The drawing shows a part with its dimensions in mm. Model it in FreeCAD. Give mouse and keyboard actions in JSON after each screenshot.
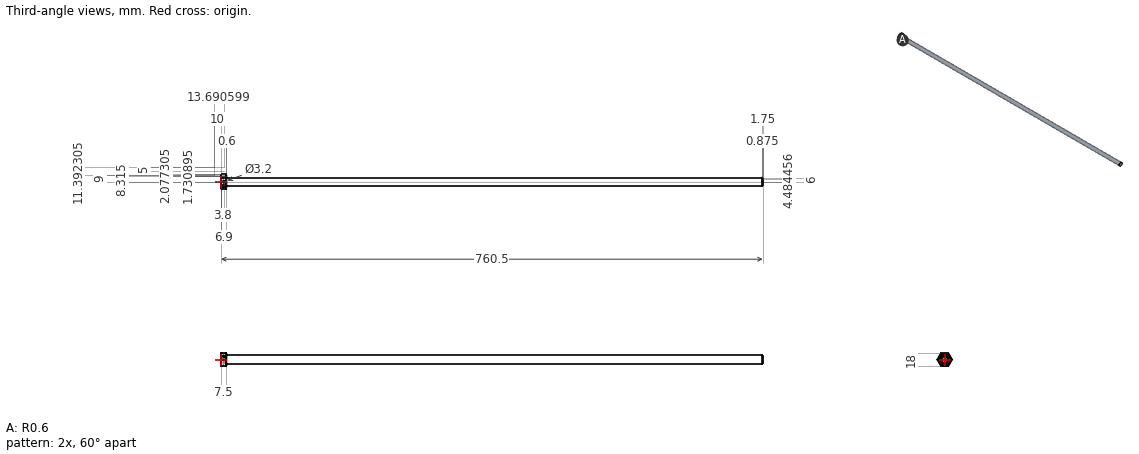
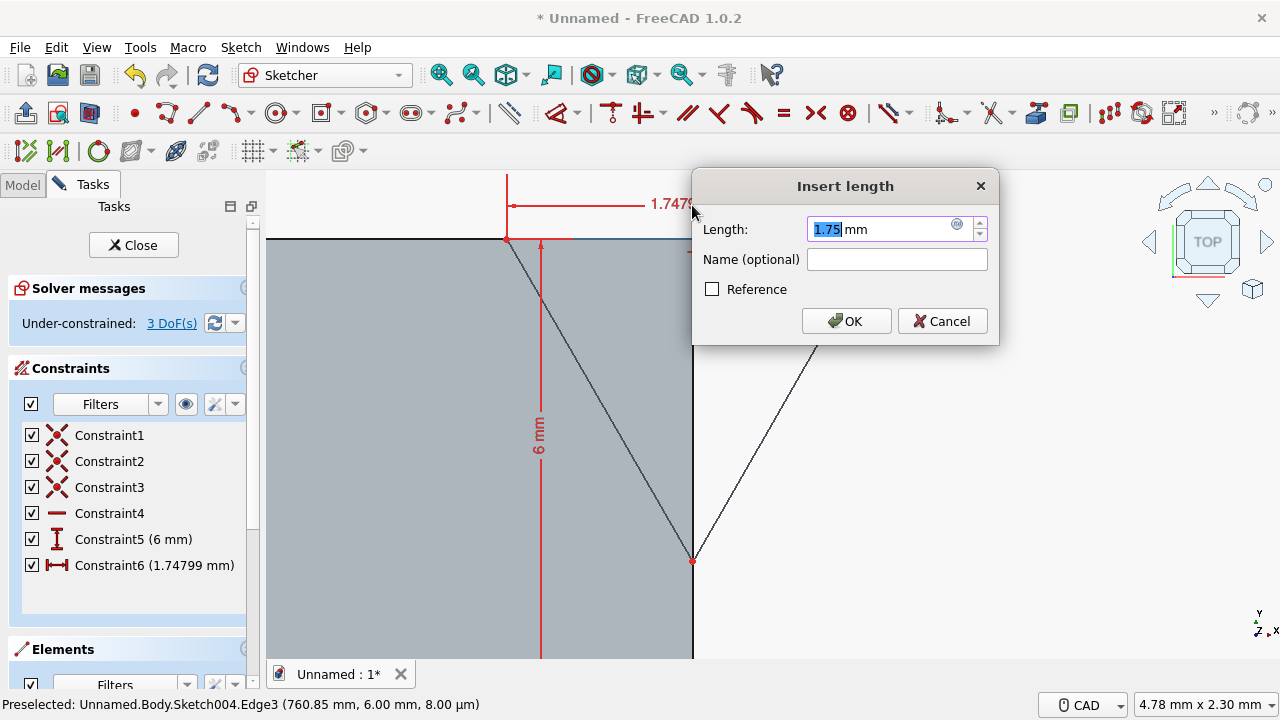
{"action": "type", "text": "1.75"}
{"action": "key", "text": "Return"}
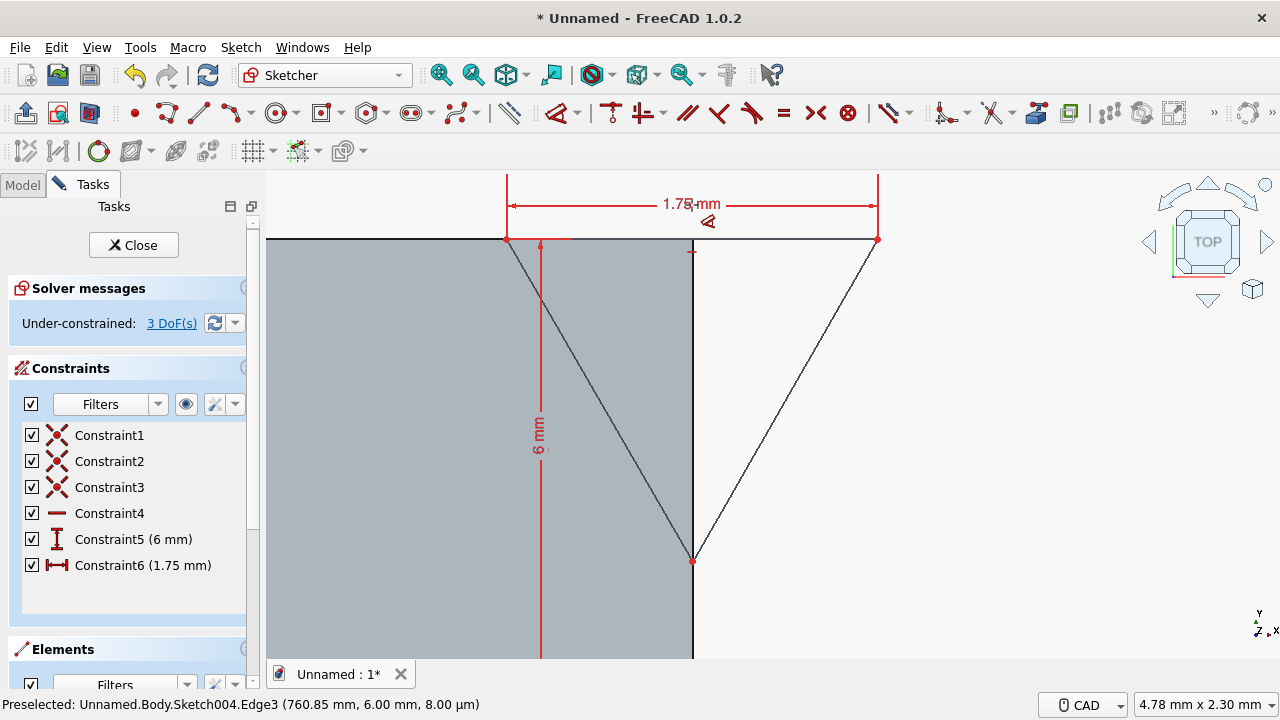
{"action": "left_click", "coordinate": [693, 562]}
{"action": "left_click", "coordinate": [493, 528]}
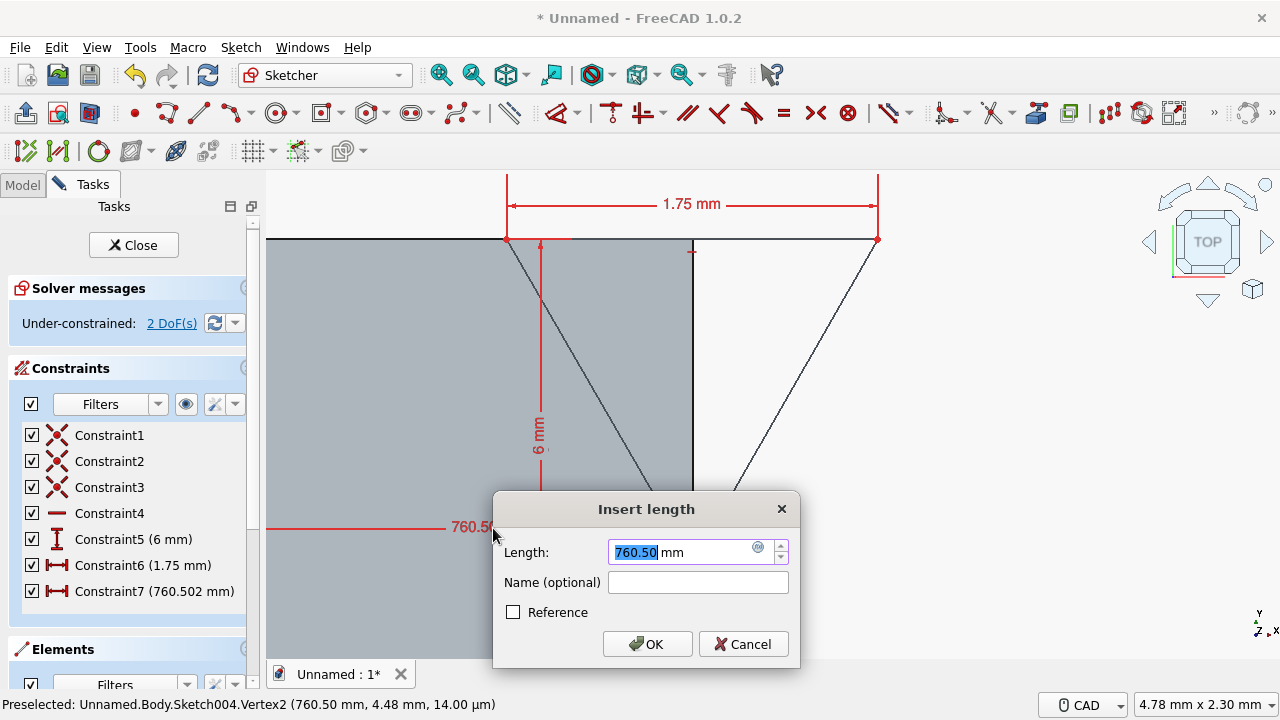
{"action": "type", "text": "760.5"}
{"action": "key", "text": "Return"}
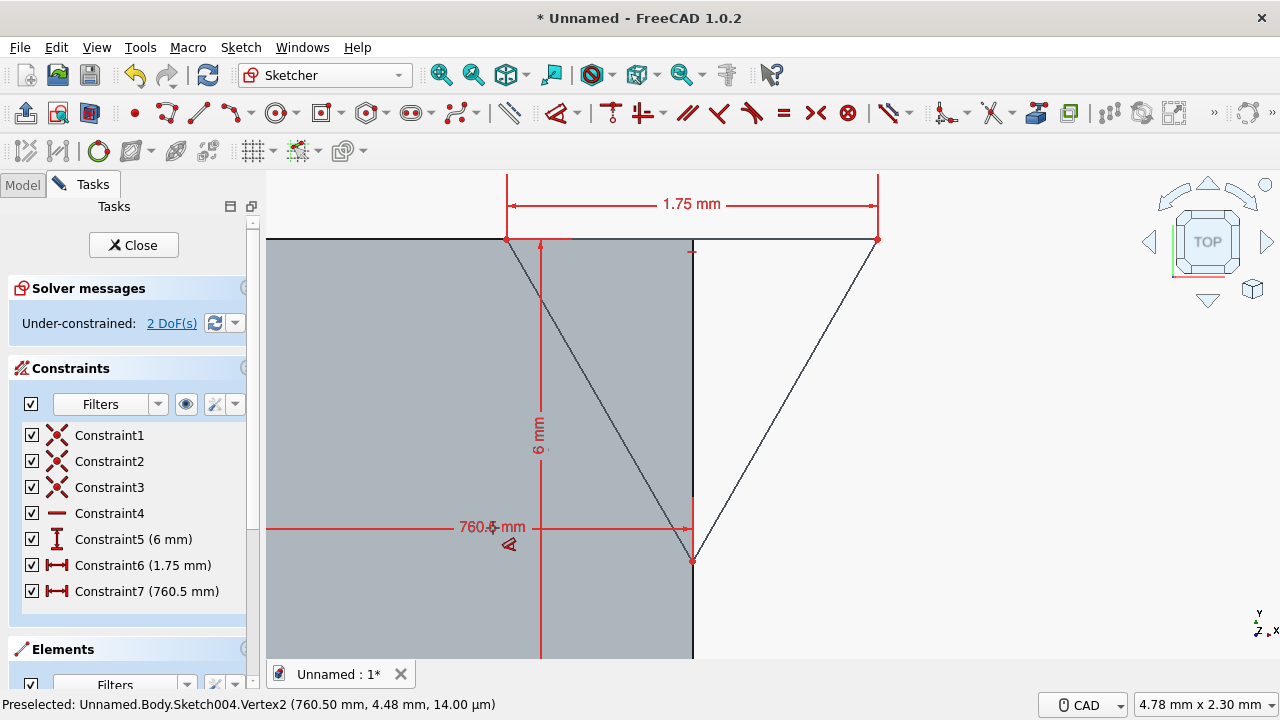
{"action": "left_click", "coordinate": [562, 336]}
{"action": "left_click", "coordinate": [600, 596]}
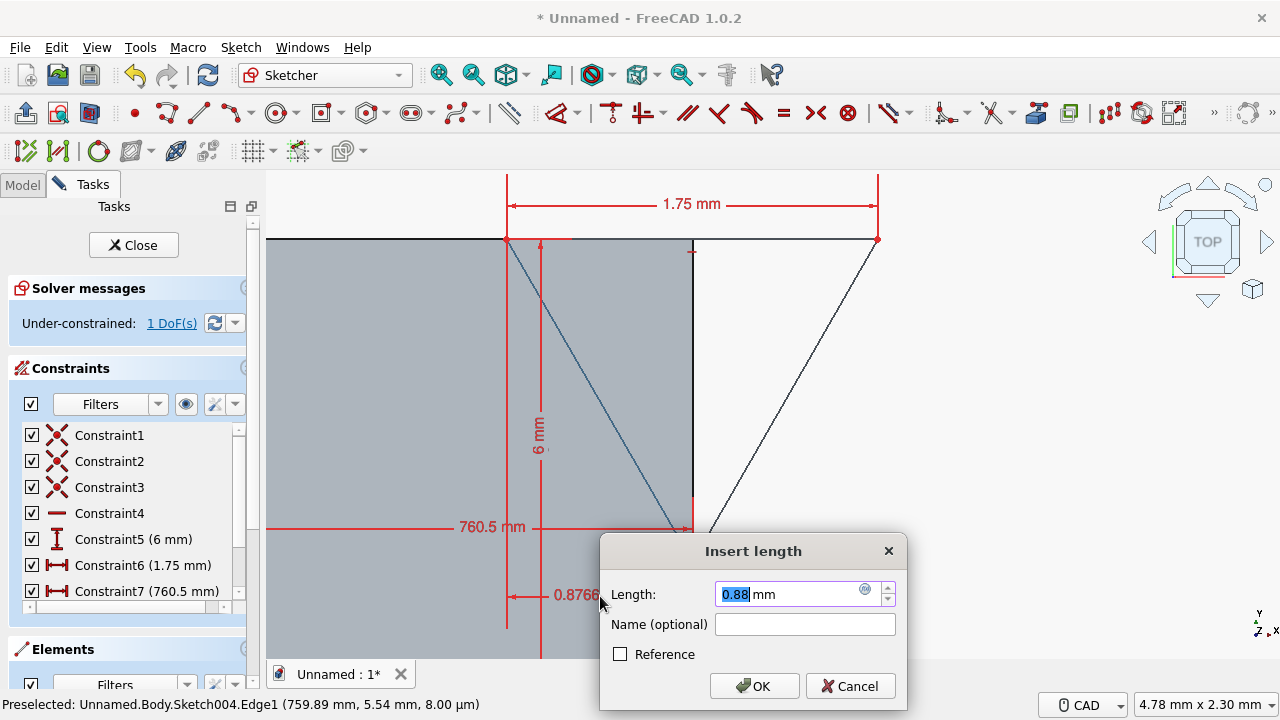
{"action": "type", "text": "0.875"}
{"action": "key", "text": "Return"}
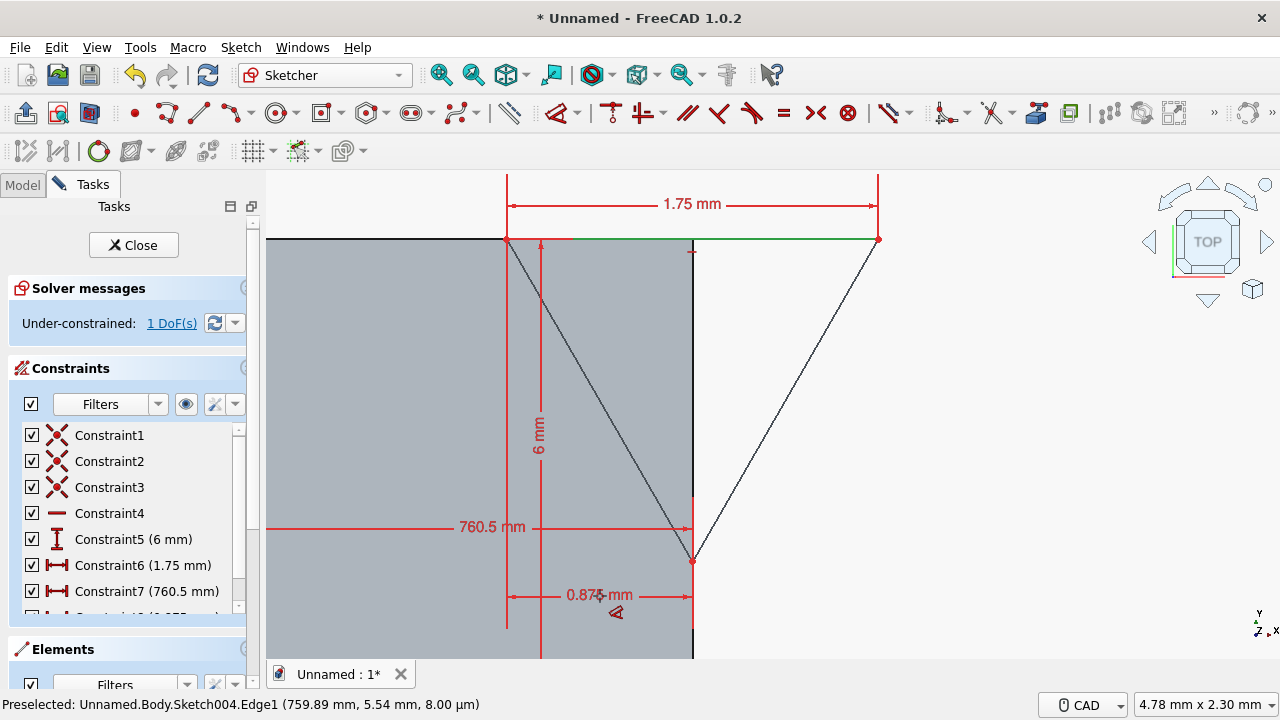
{"action": "left_click", "coordinate": [693, 562]}
{"action": "left_click", "coordinate": [727, 596]}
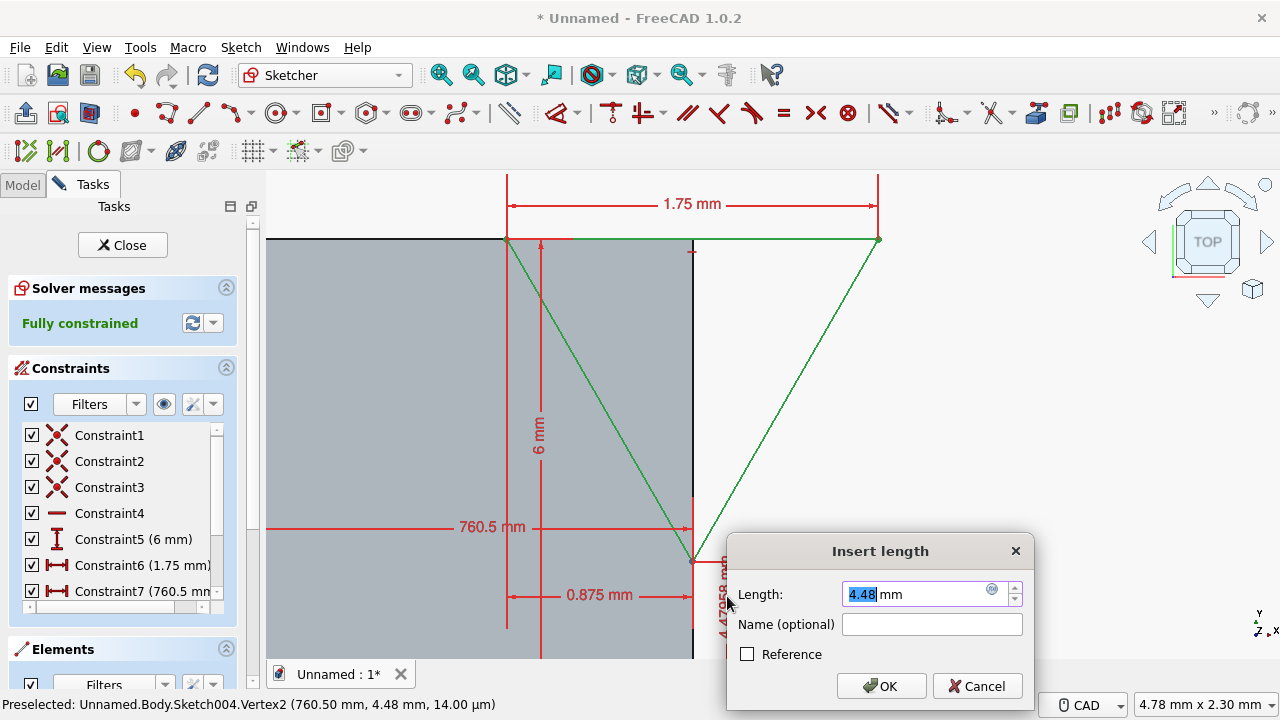
{"action": "type", "text": "4.484456"}
{"action": "key", "text": "Return"}
{"action": "key", "text": "Escape"}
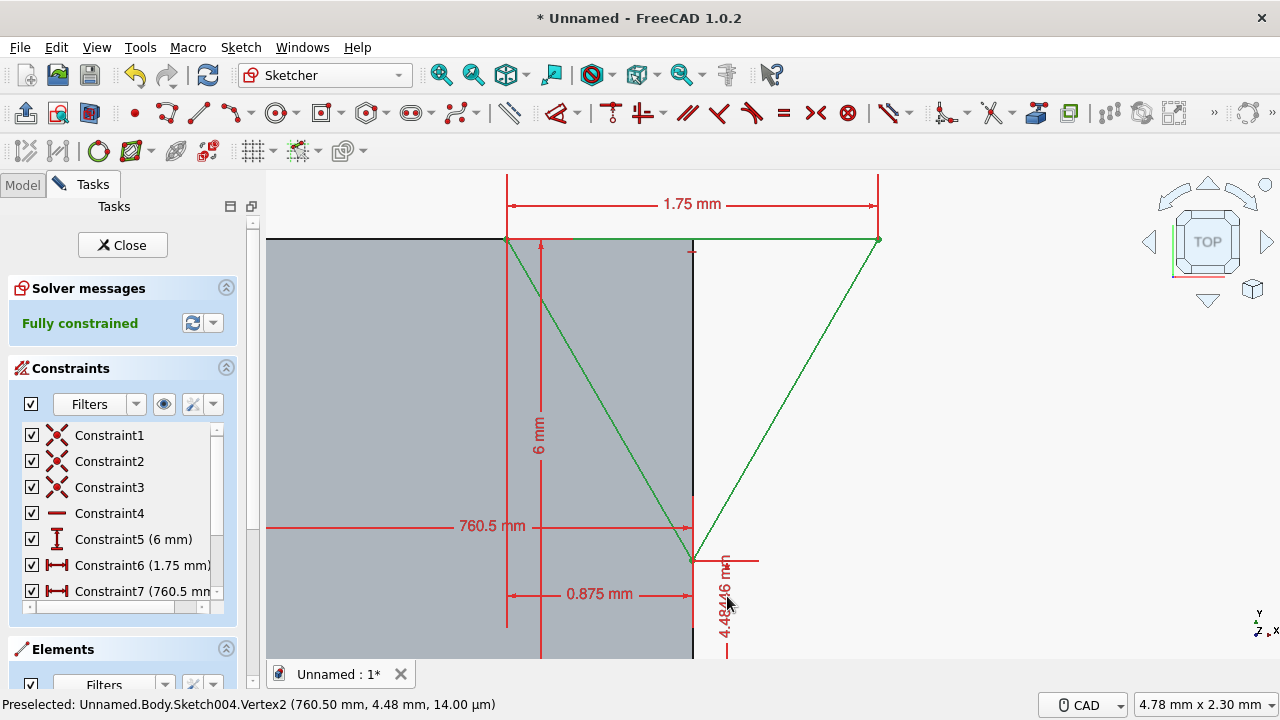
{"action": "left_click", "coordinate": [123, 245]}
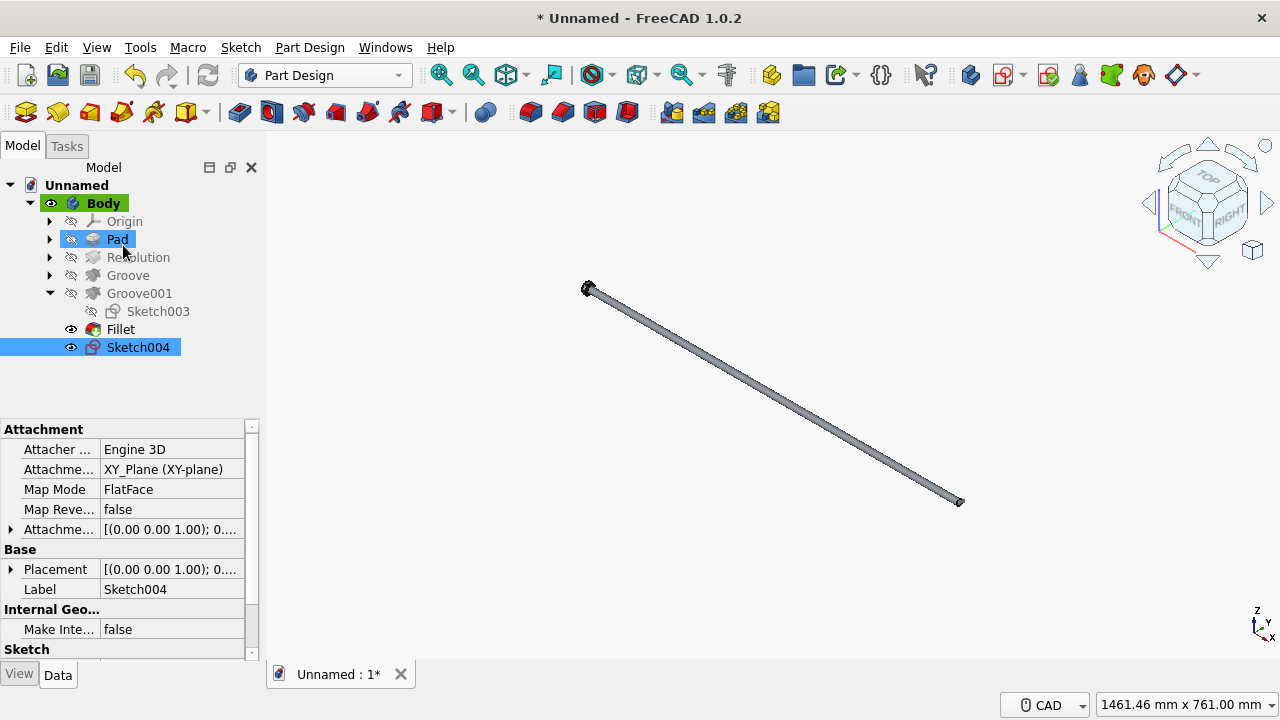
{"action": "left_click", "coordinate": [304, 112]}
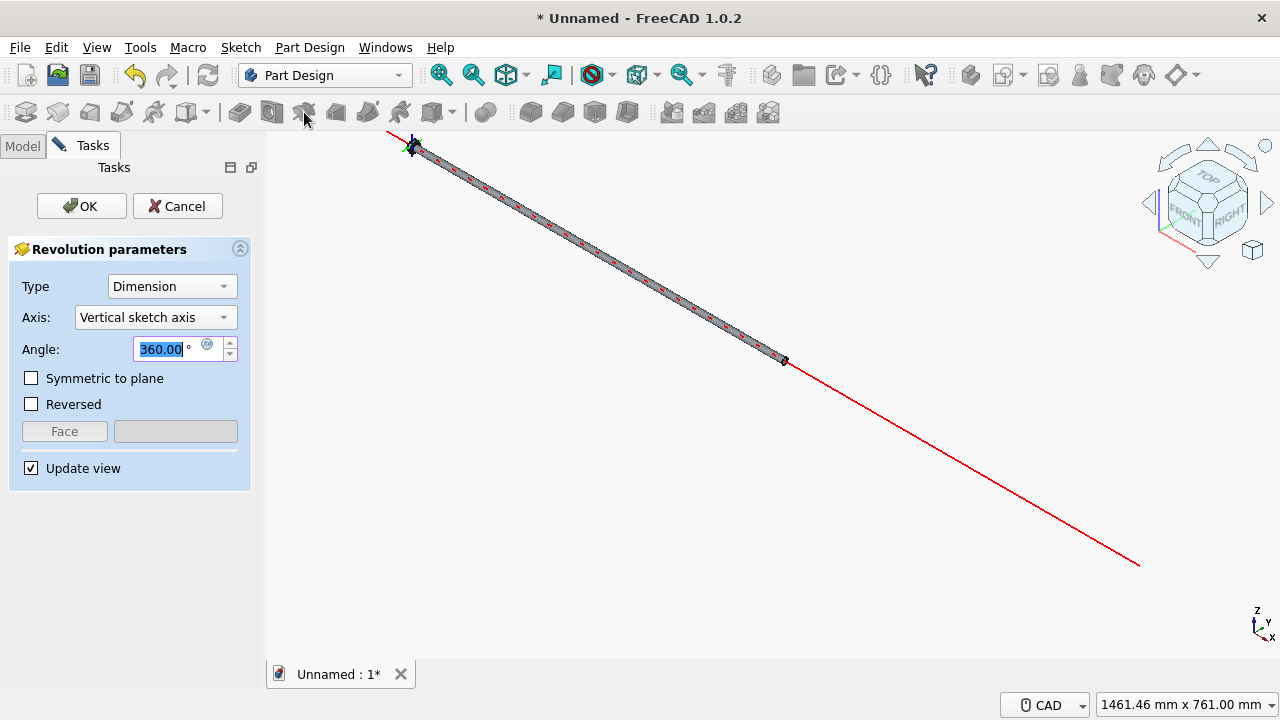
{"action": "left_click", "coordinate": [156, 318]}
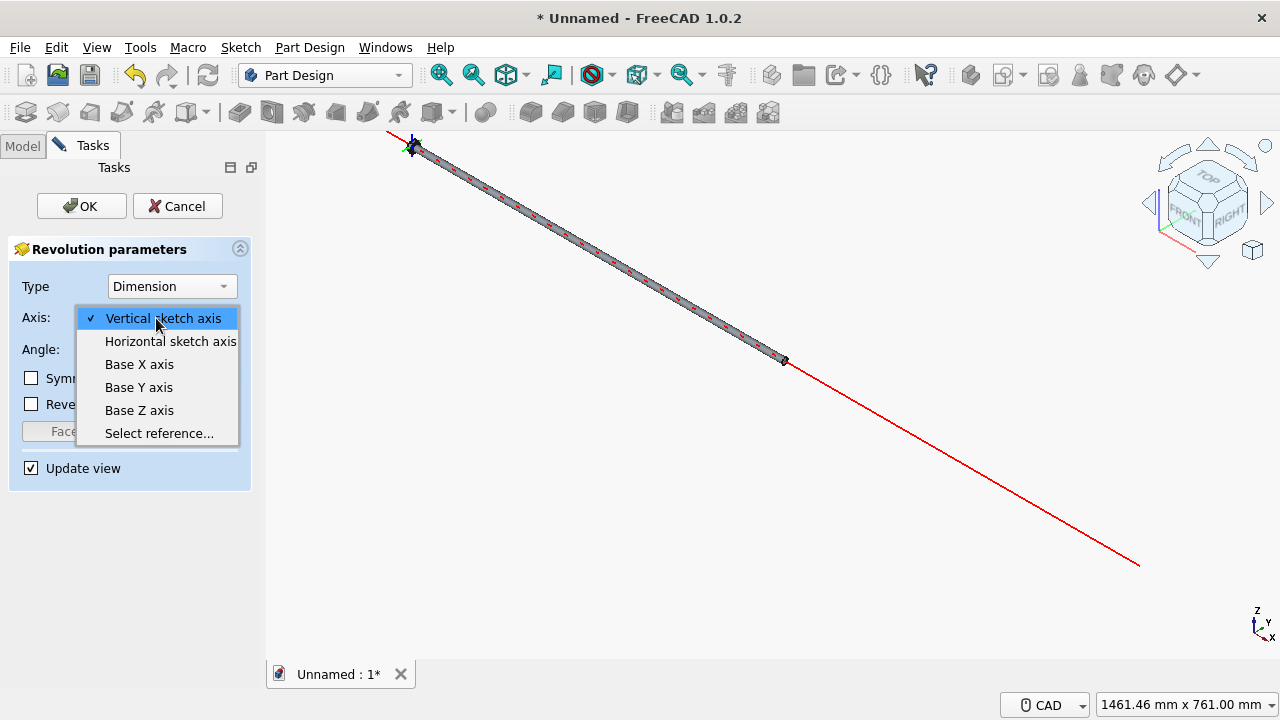
{"action": "left_click", "coordinate": [156, 342]}